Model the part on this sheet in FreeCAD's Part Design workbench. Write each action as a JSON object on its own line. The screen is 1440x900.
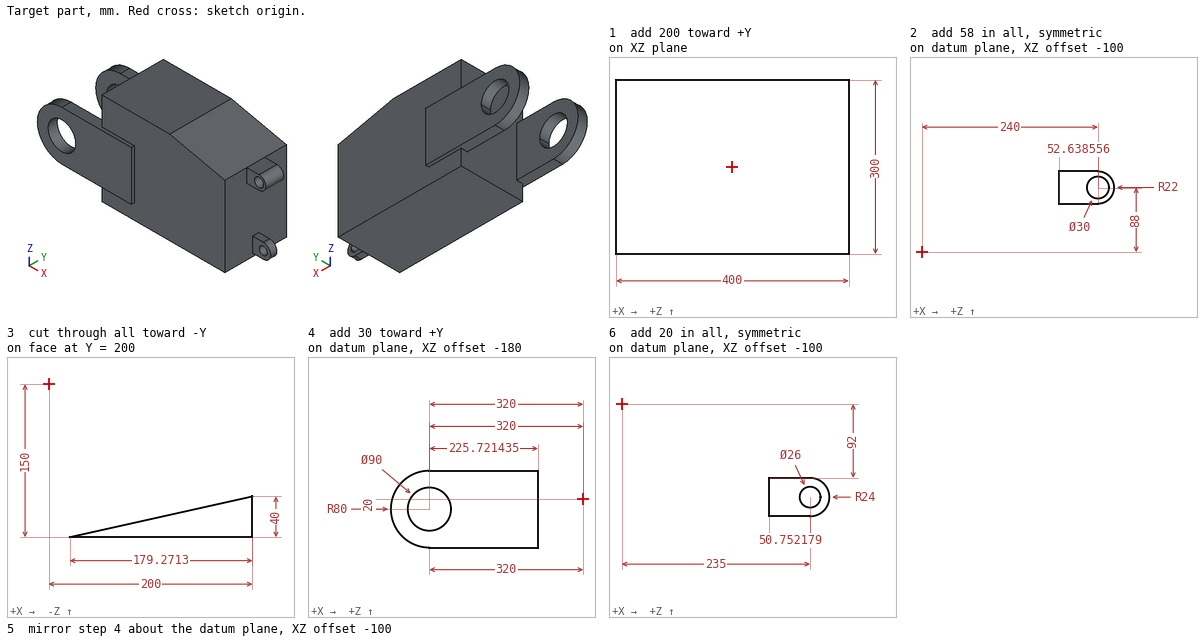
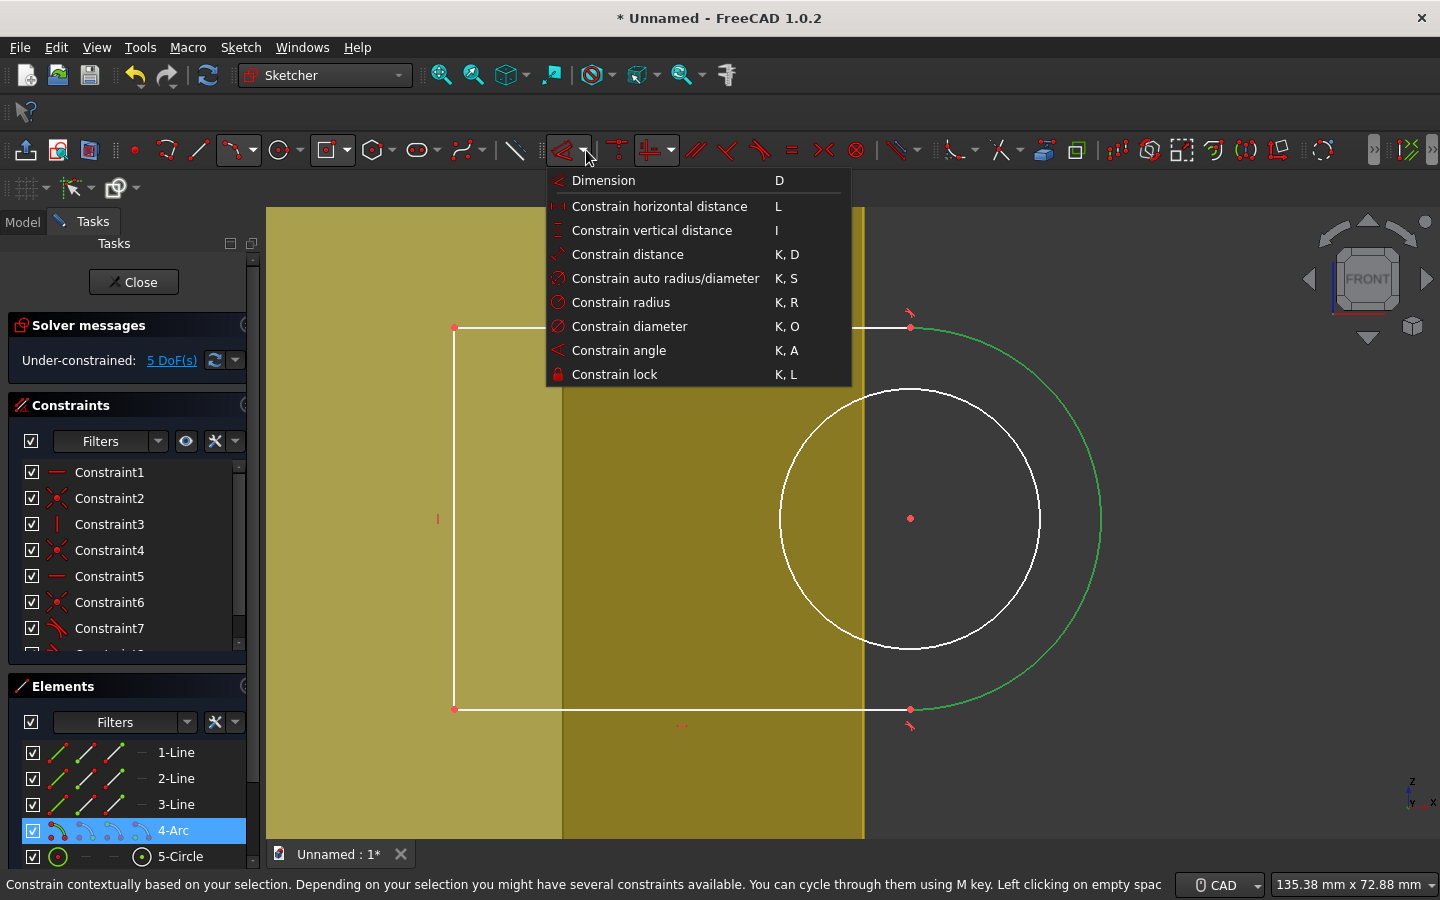
{"action": "left_click", "coordinate": [699, 302]}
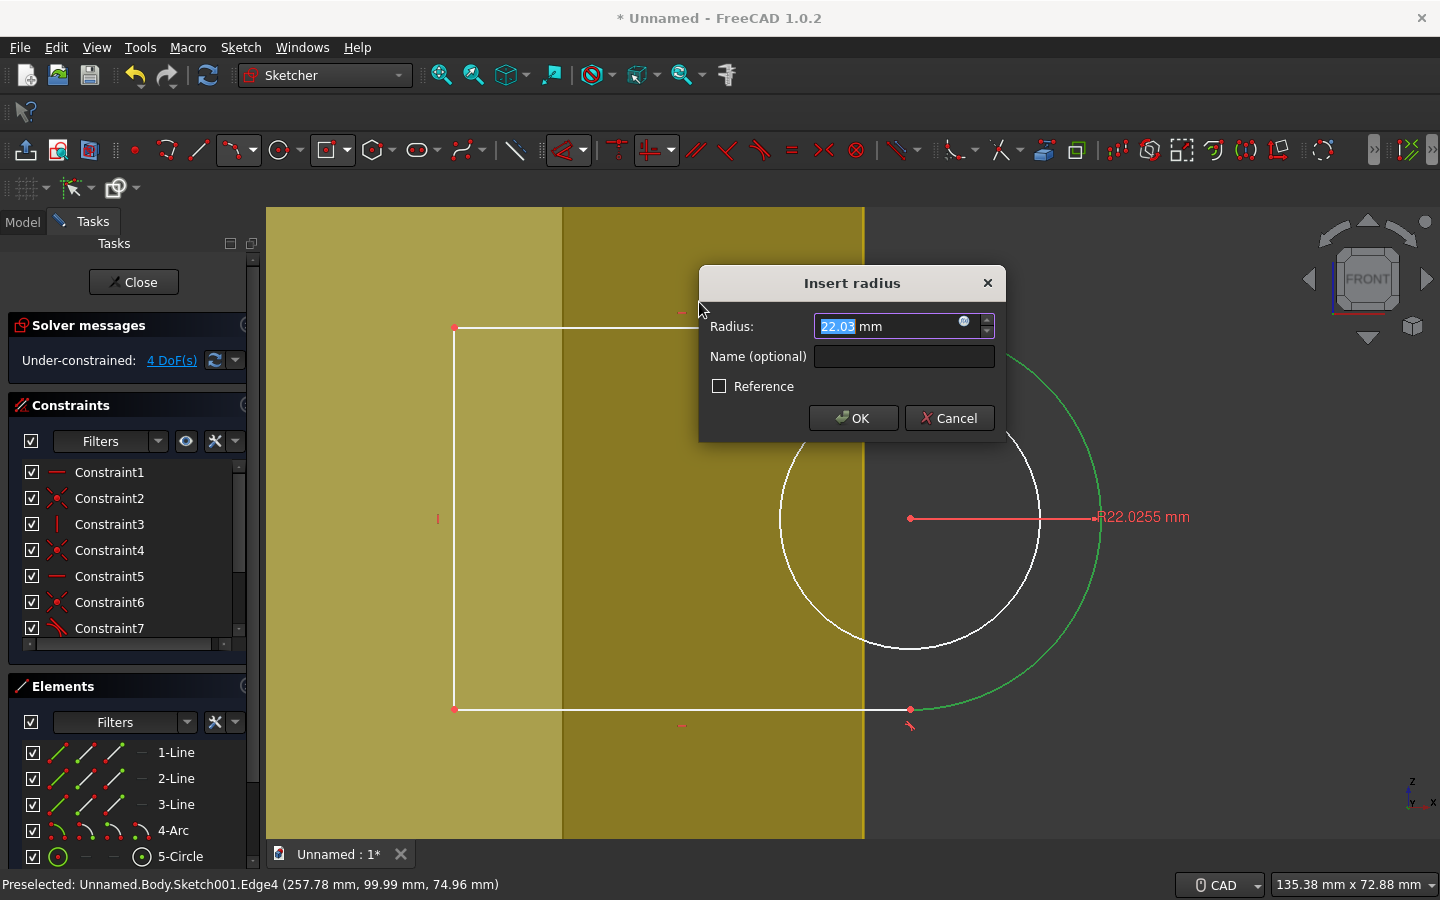
{"action": "type", "text": "22"}
{"action": "key", "text": "Return"}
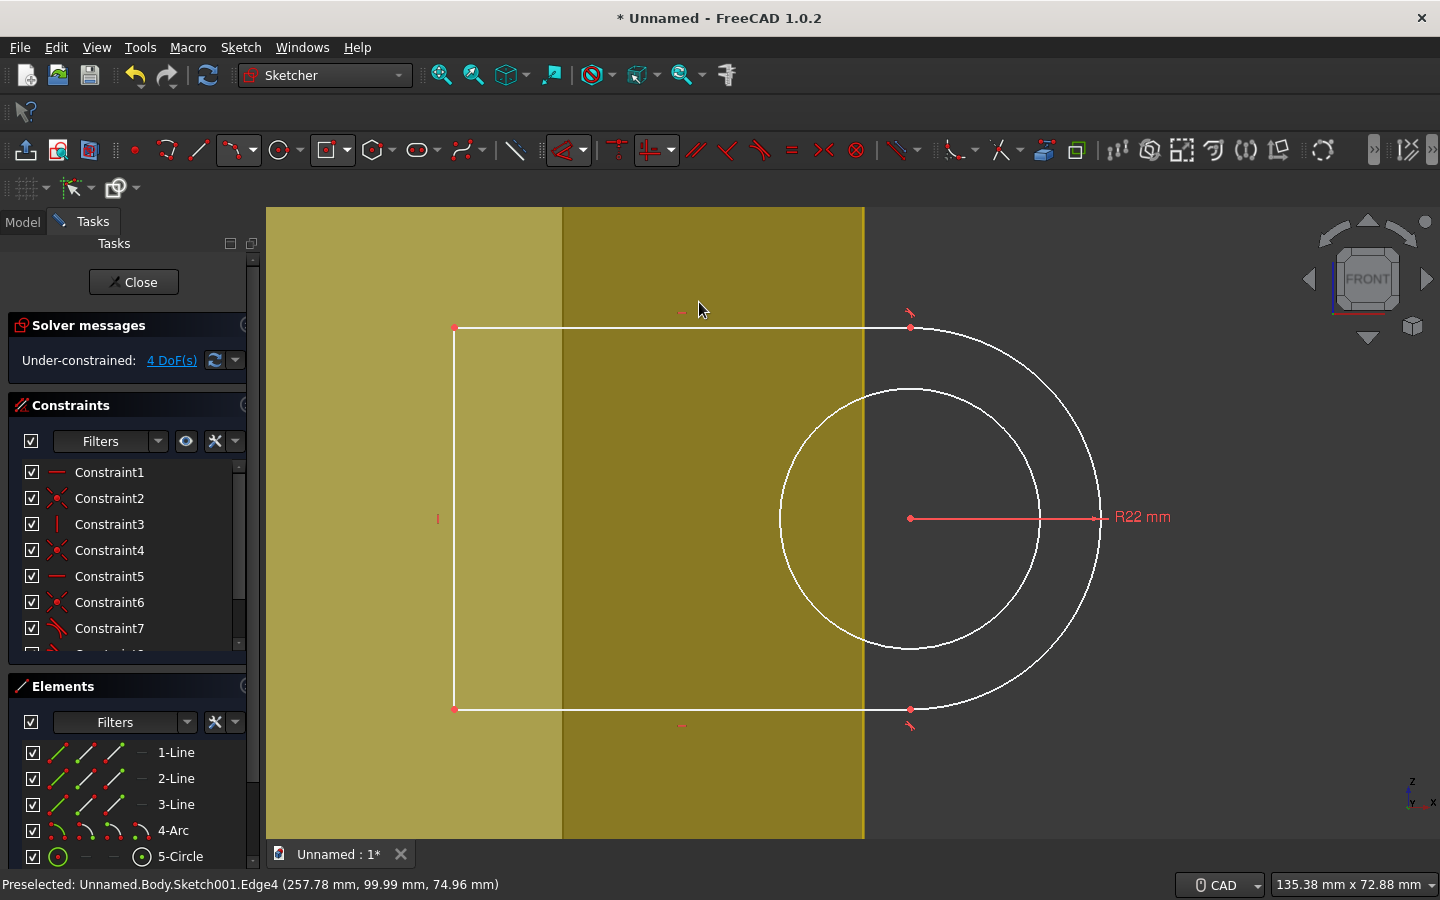
{"action": "left_click", "coordinate": [1002, 426]}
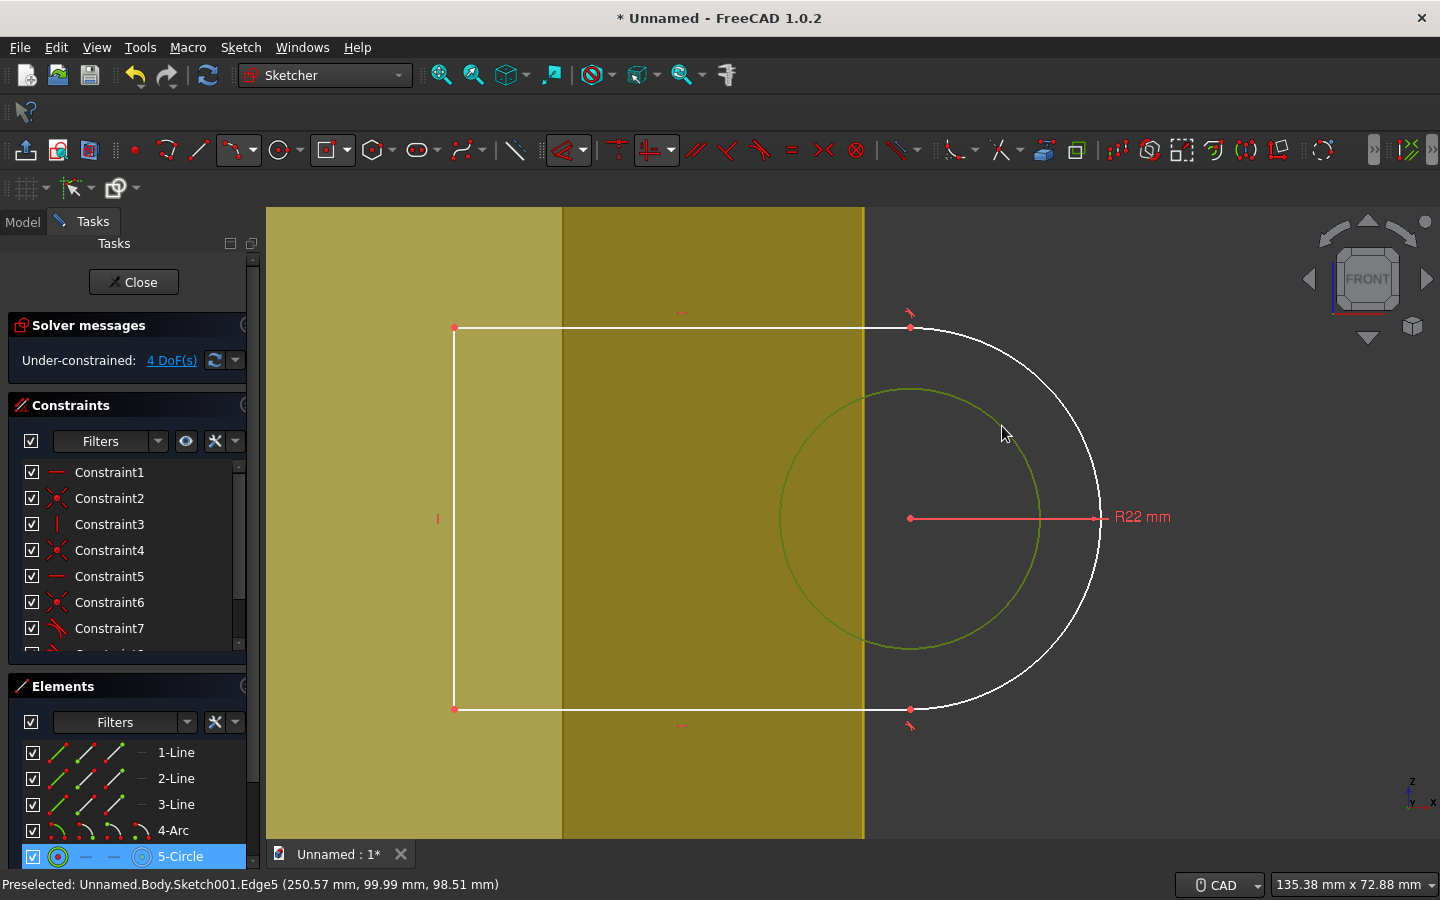
{"action": "left_click", "coordinate": [586, 150]}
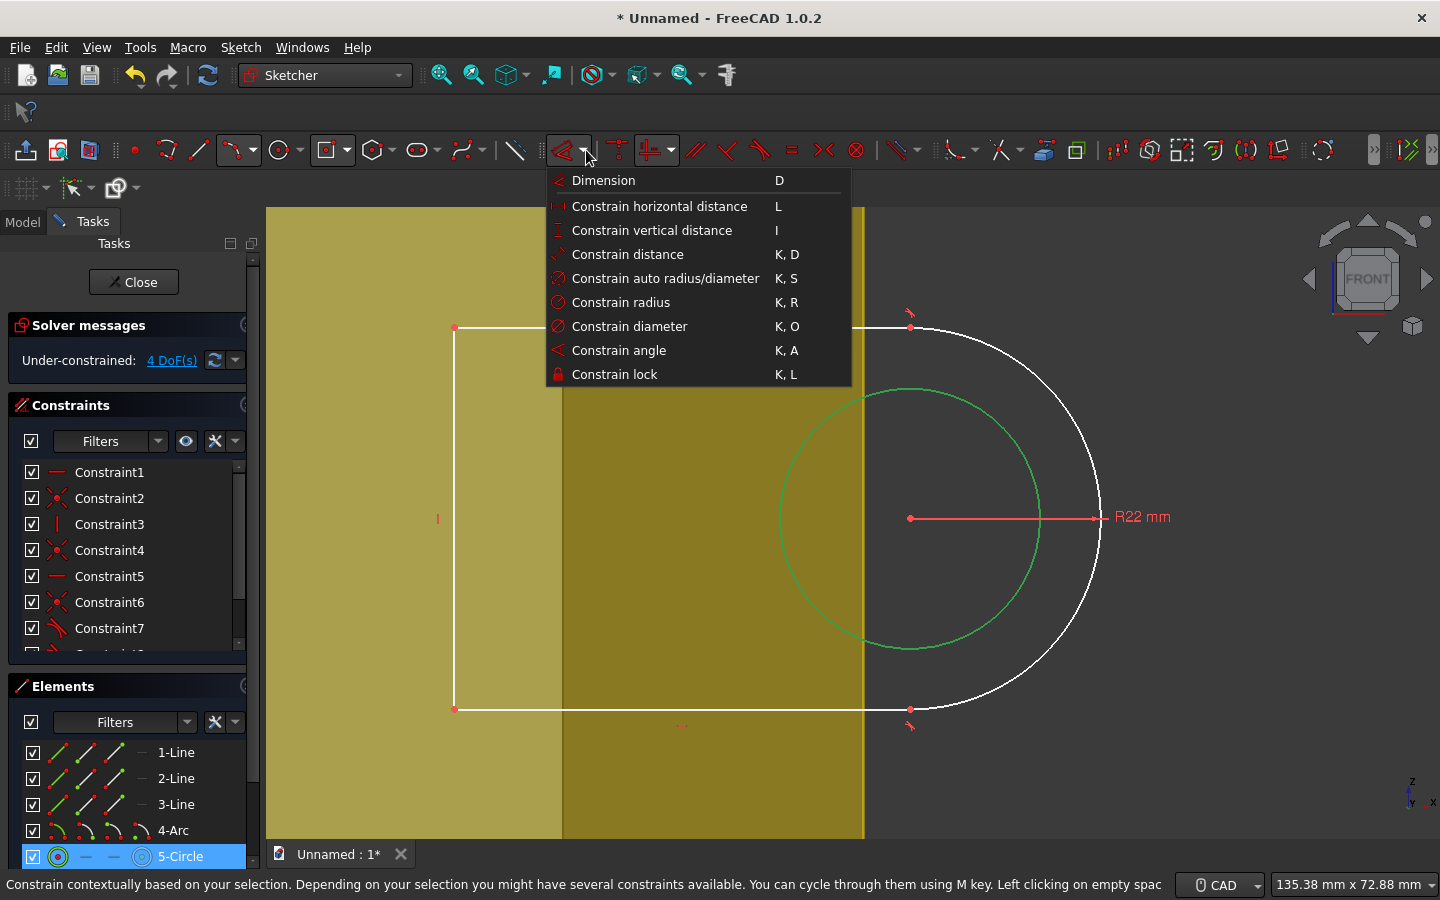
{"action": "left_click", "coordinate": [699, 326]}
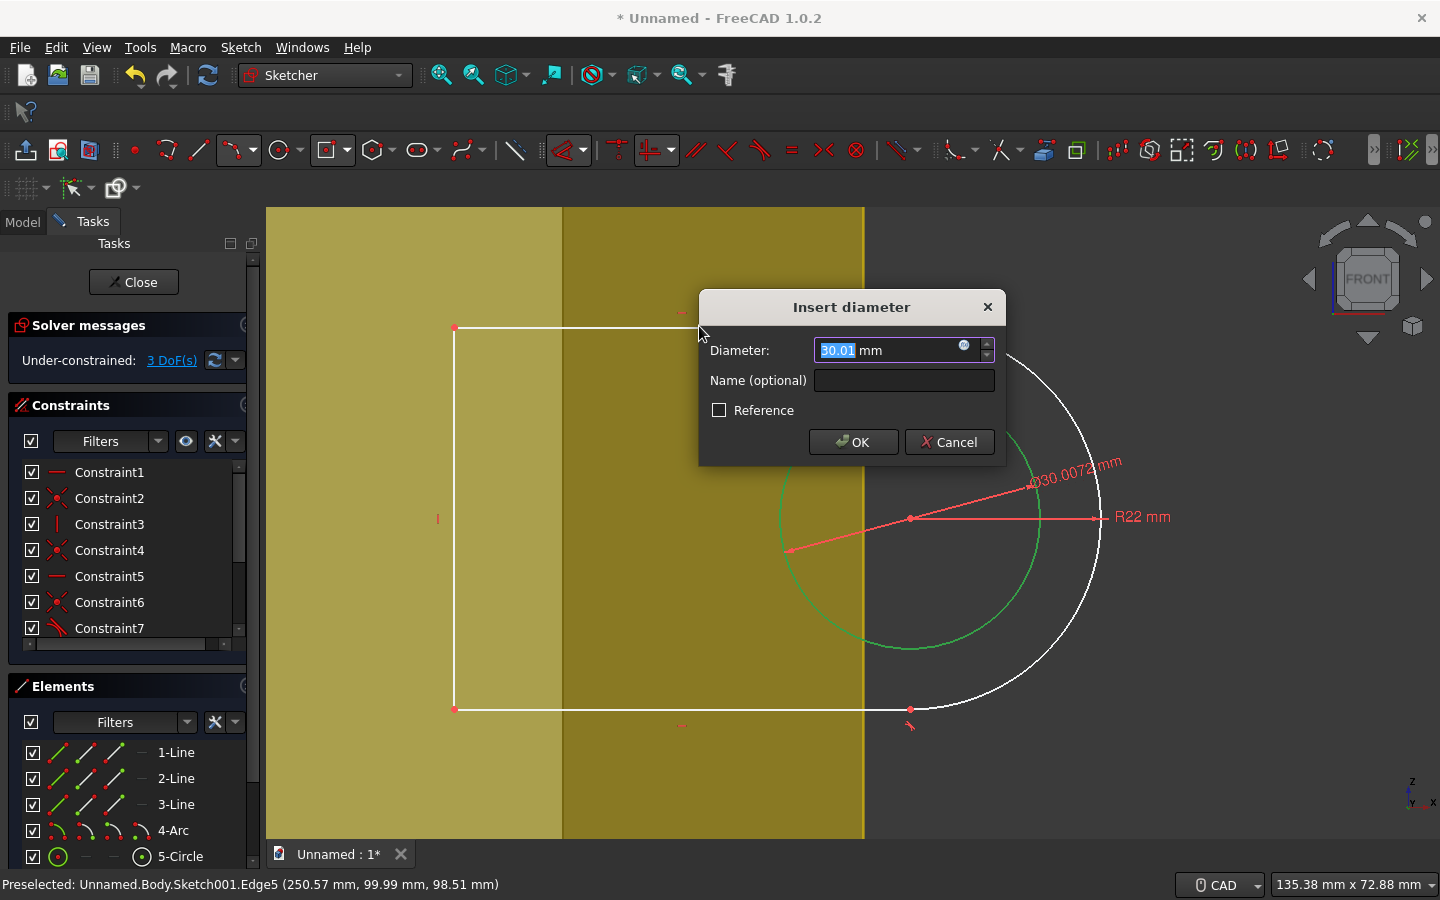
{"action": "type", "text": "30"}
{"action": "key", "text": "Return"}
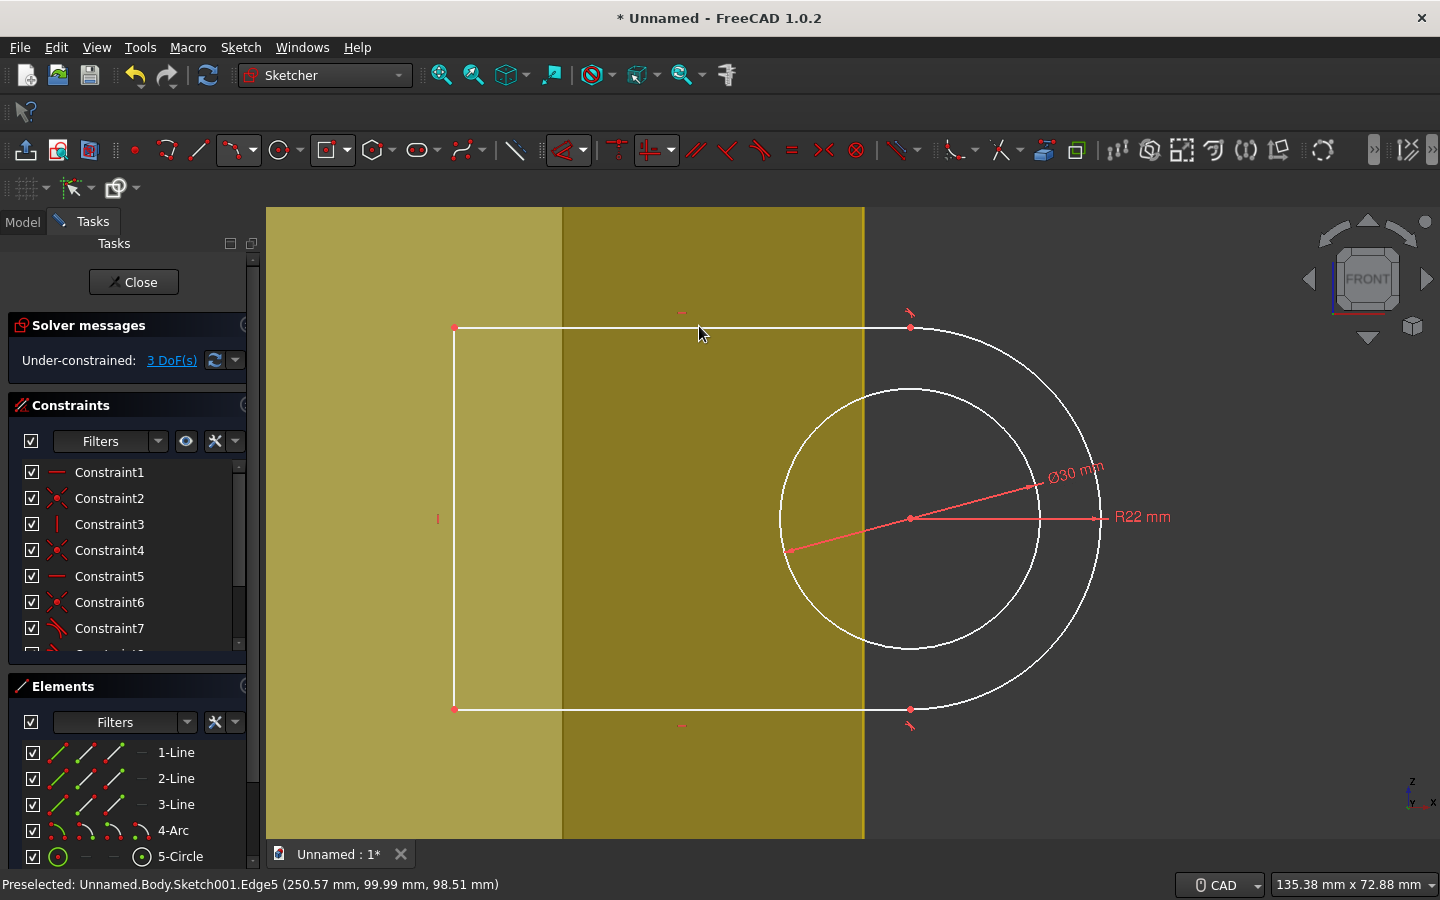
{"action": "left_click", "coordinate": [910, 519]}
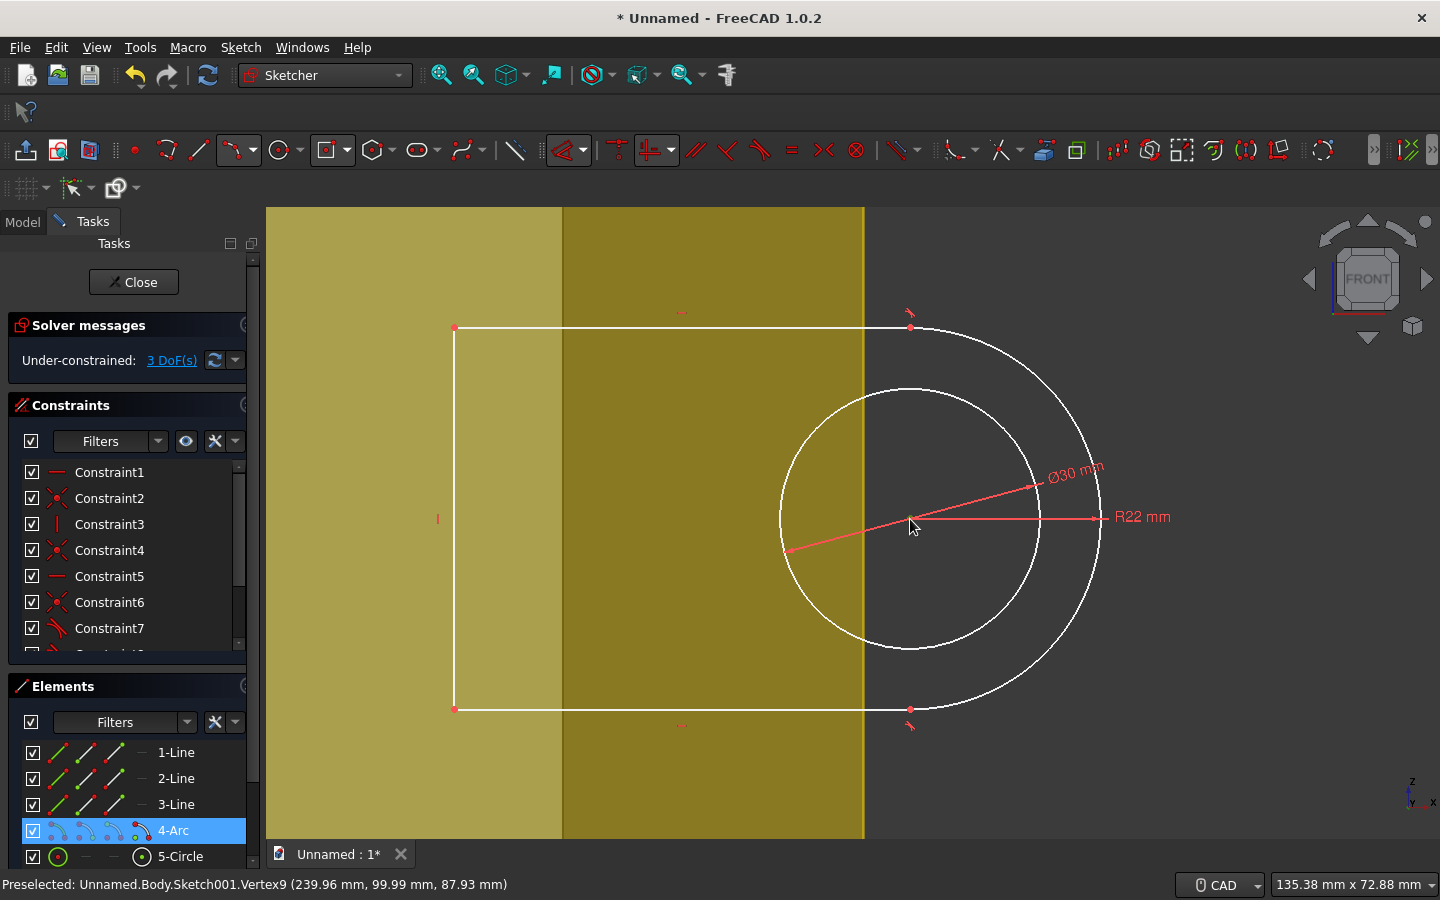
{"action": "key", "text": "i"}